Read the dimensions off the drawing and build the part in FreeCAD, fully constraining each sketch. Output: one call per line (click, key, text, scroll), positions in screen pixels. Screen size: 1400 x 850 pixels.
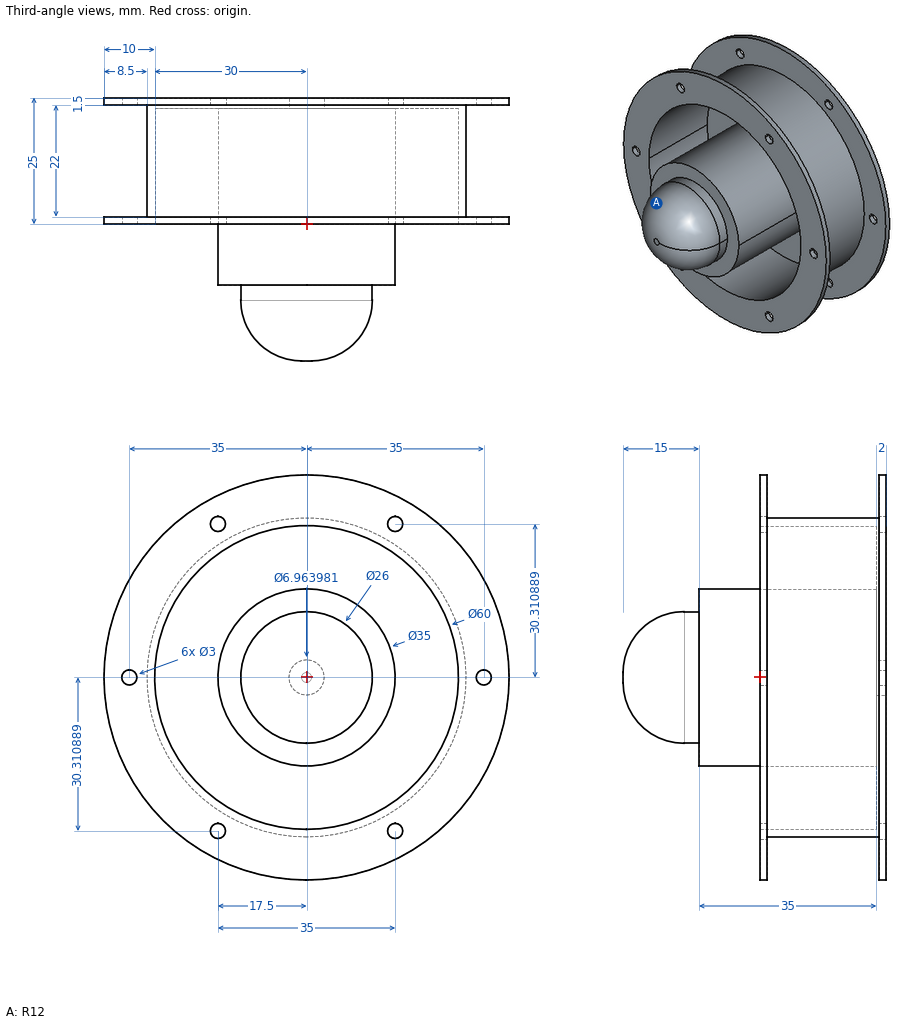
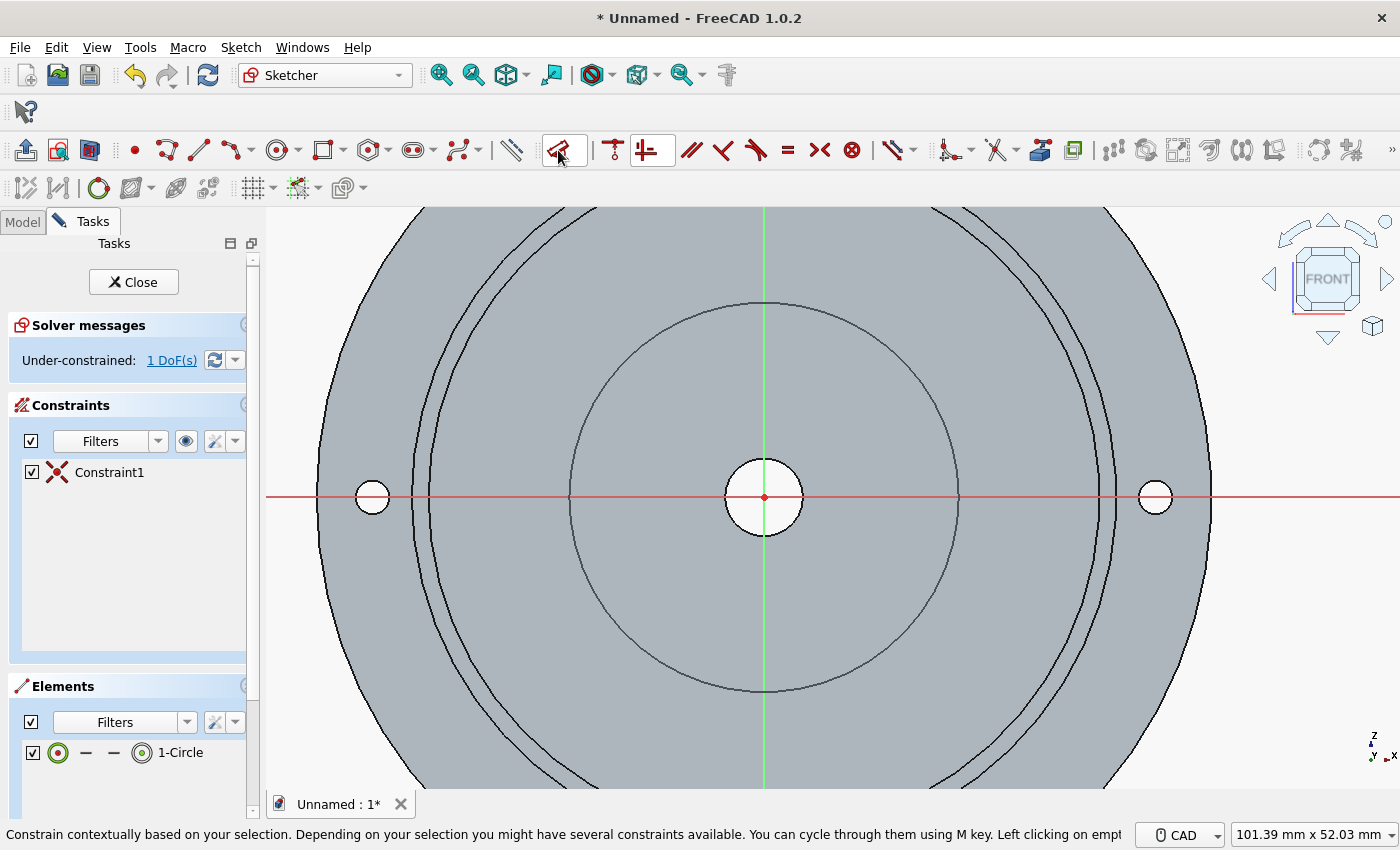
click(901, 359)
click(924, 336)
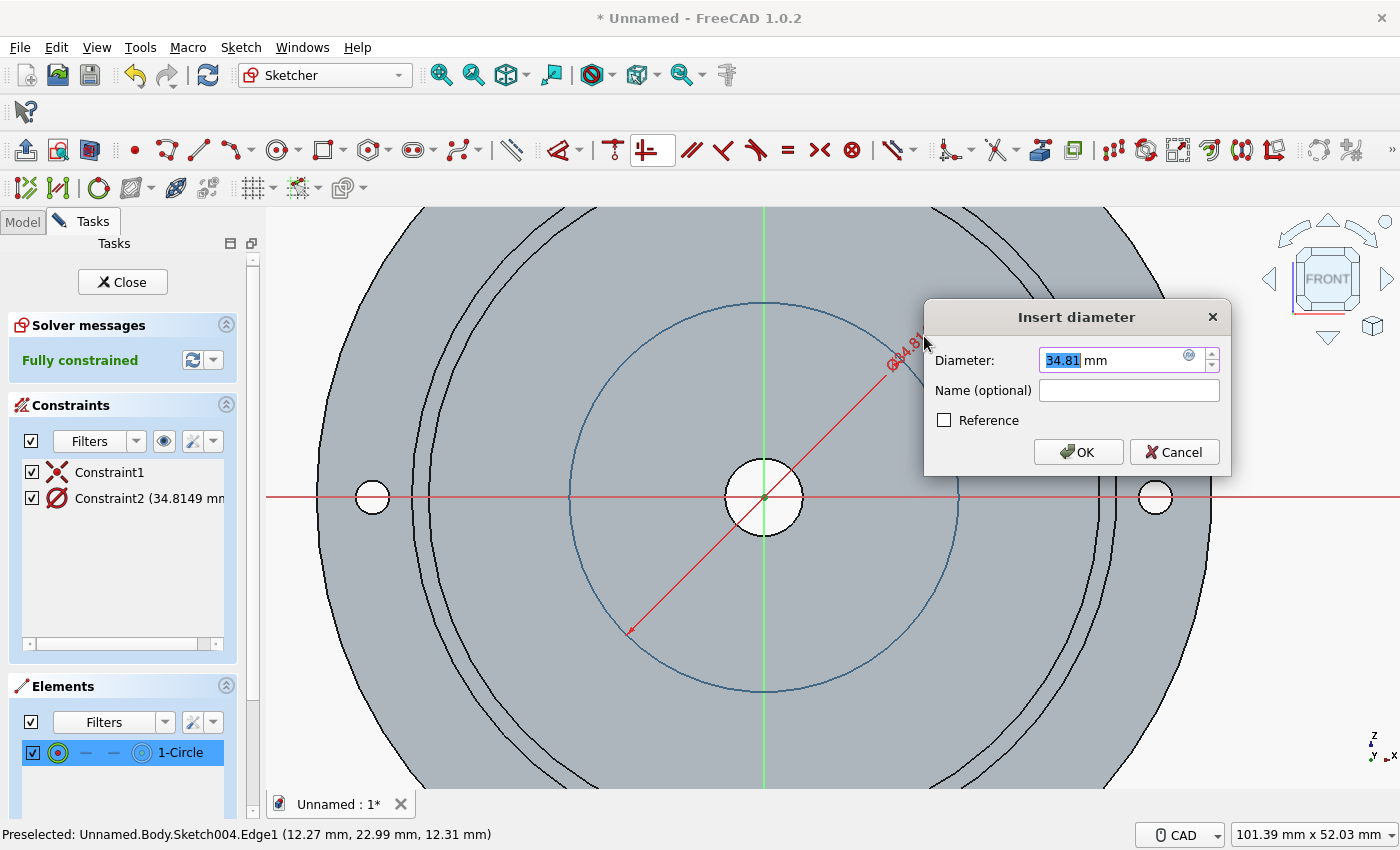
text(35)
key(Return)
key(Escape)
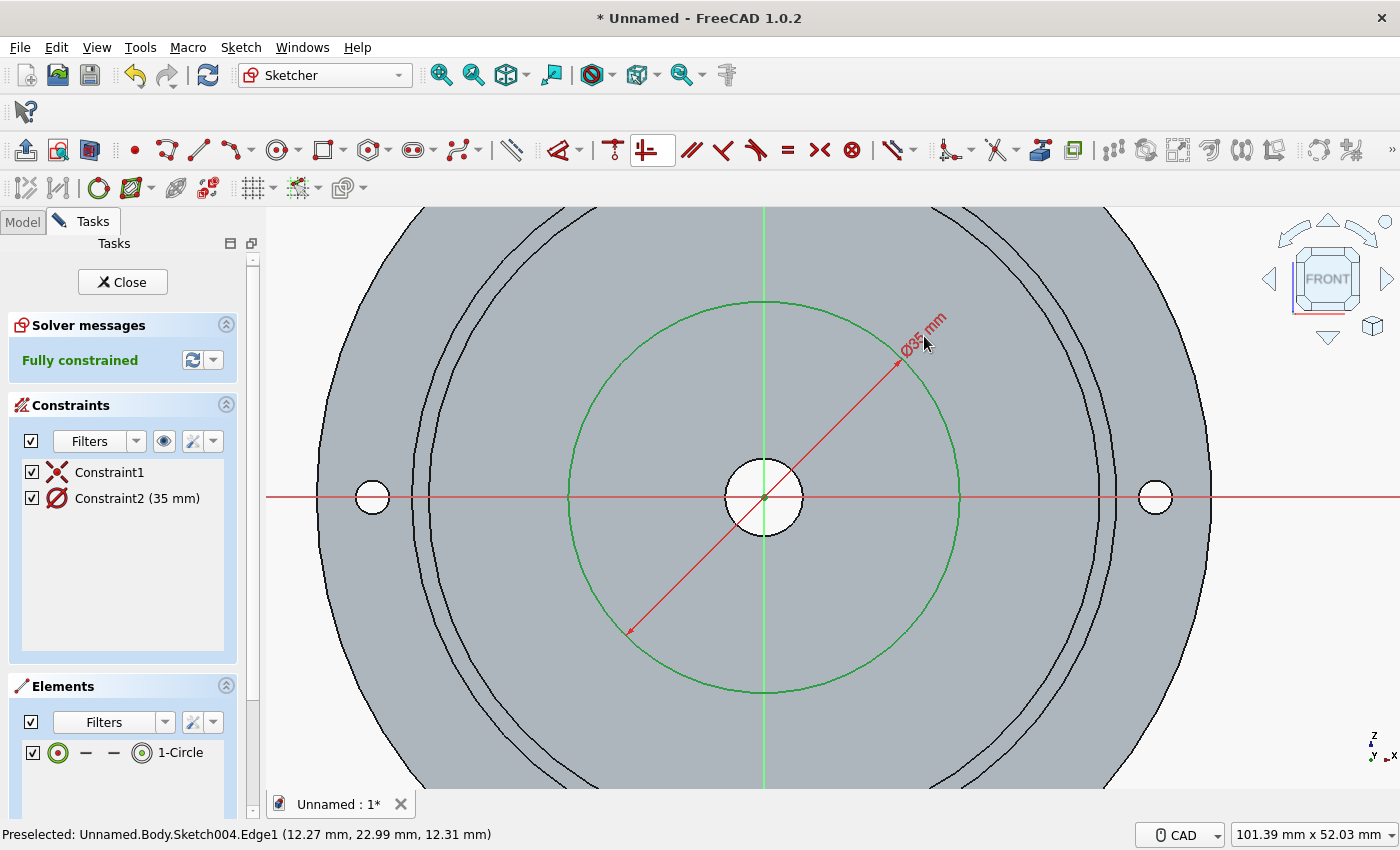
click(123, 282)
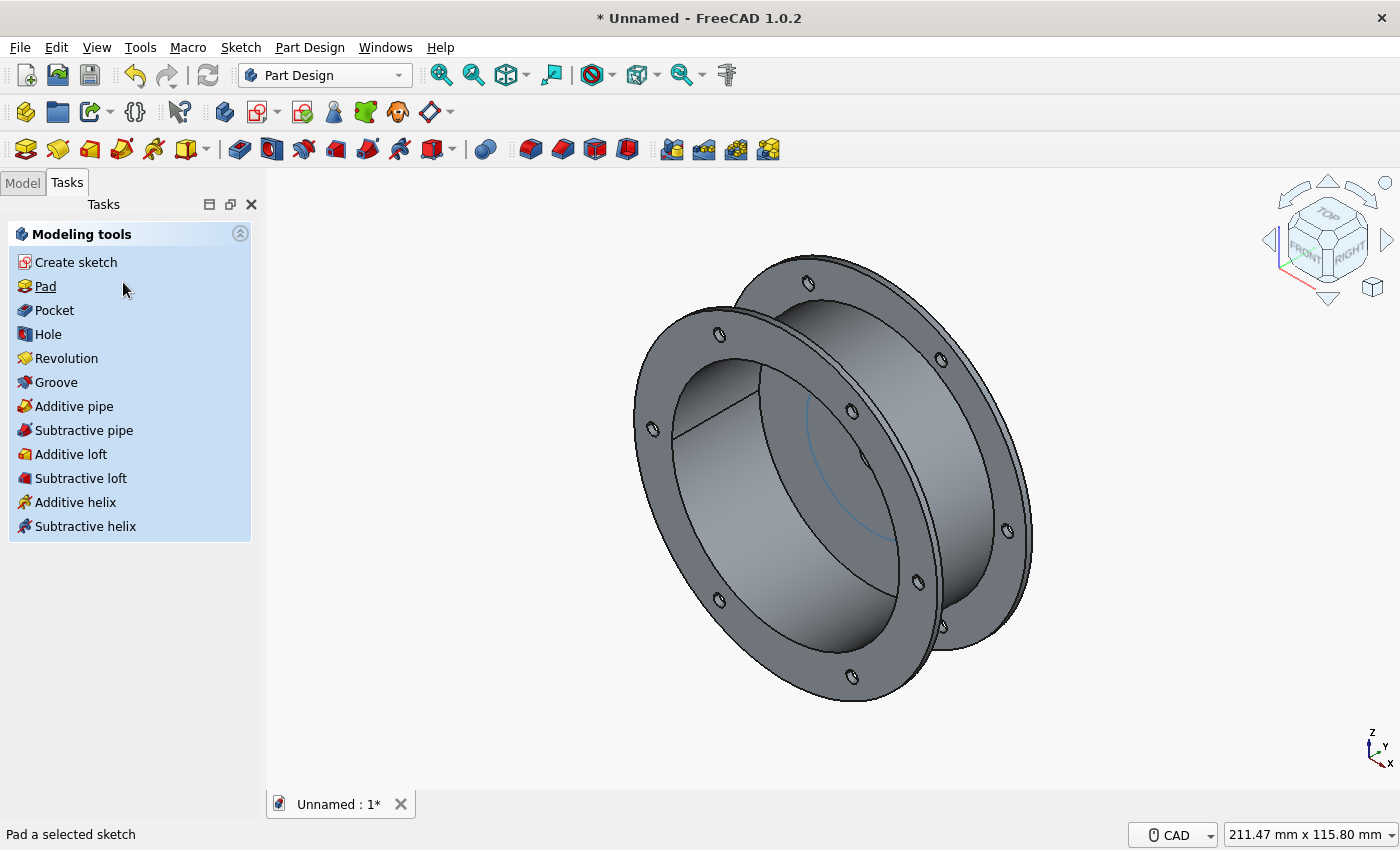
click(26, 150)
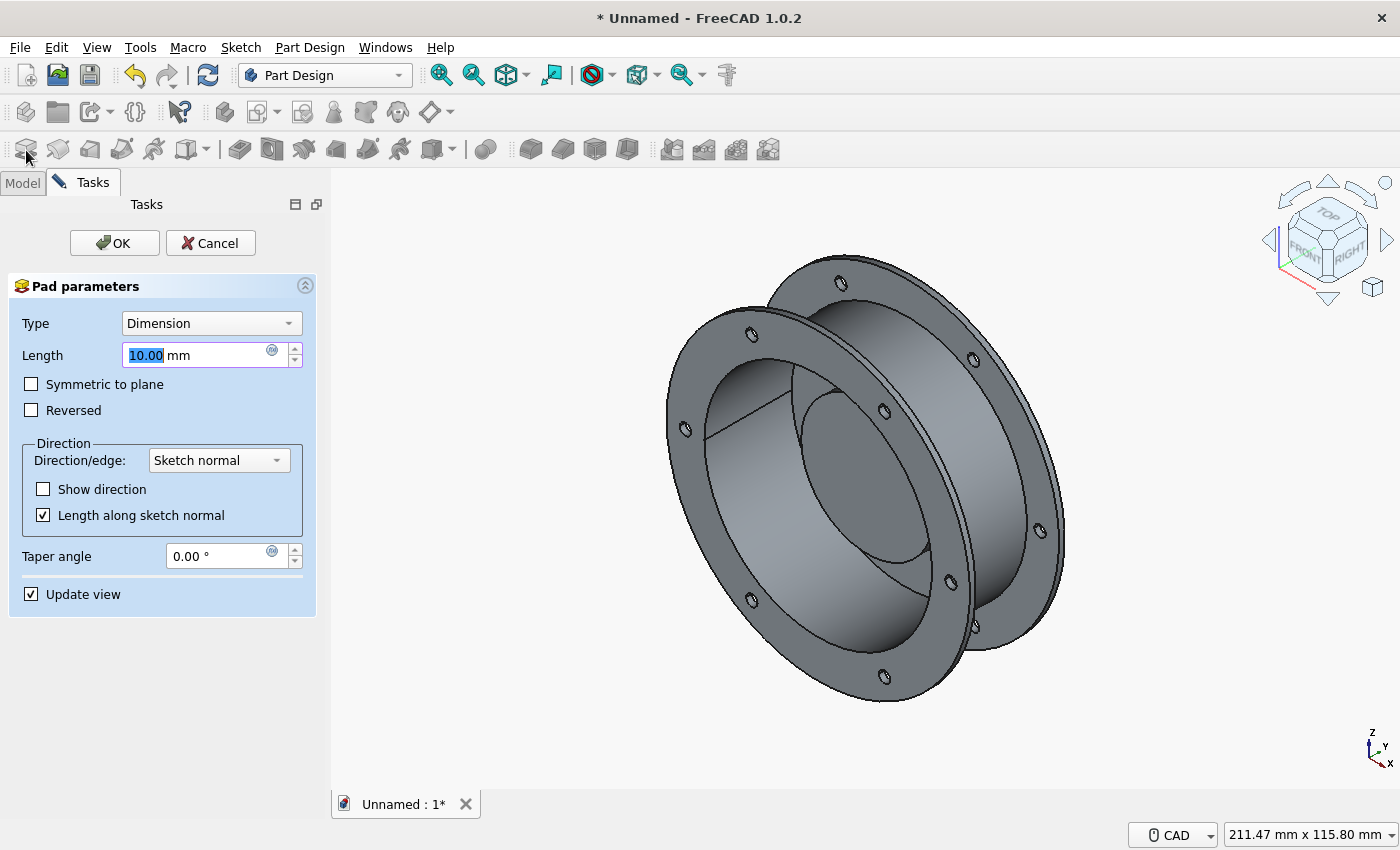
text(35)
key(Tab)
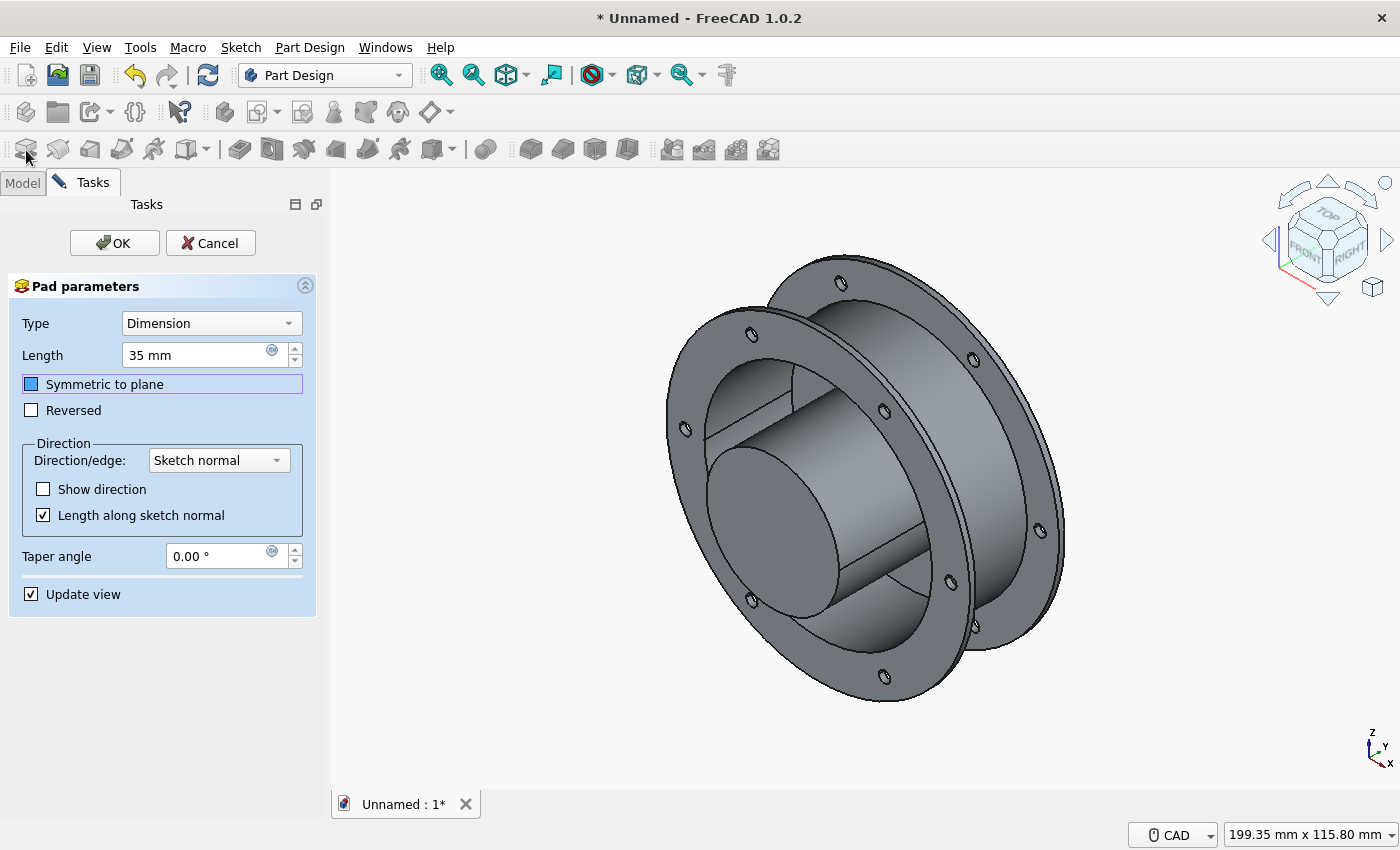
click(115, 243)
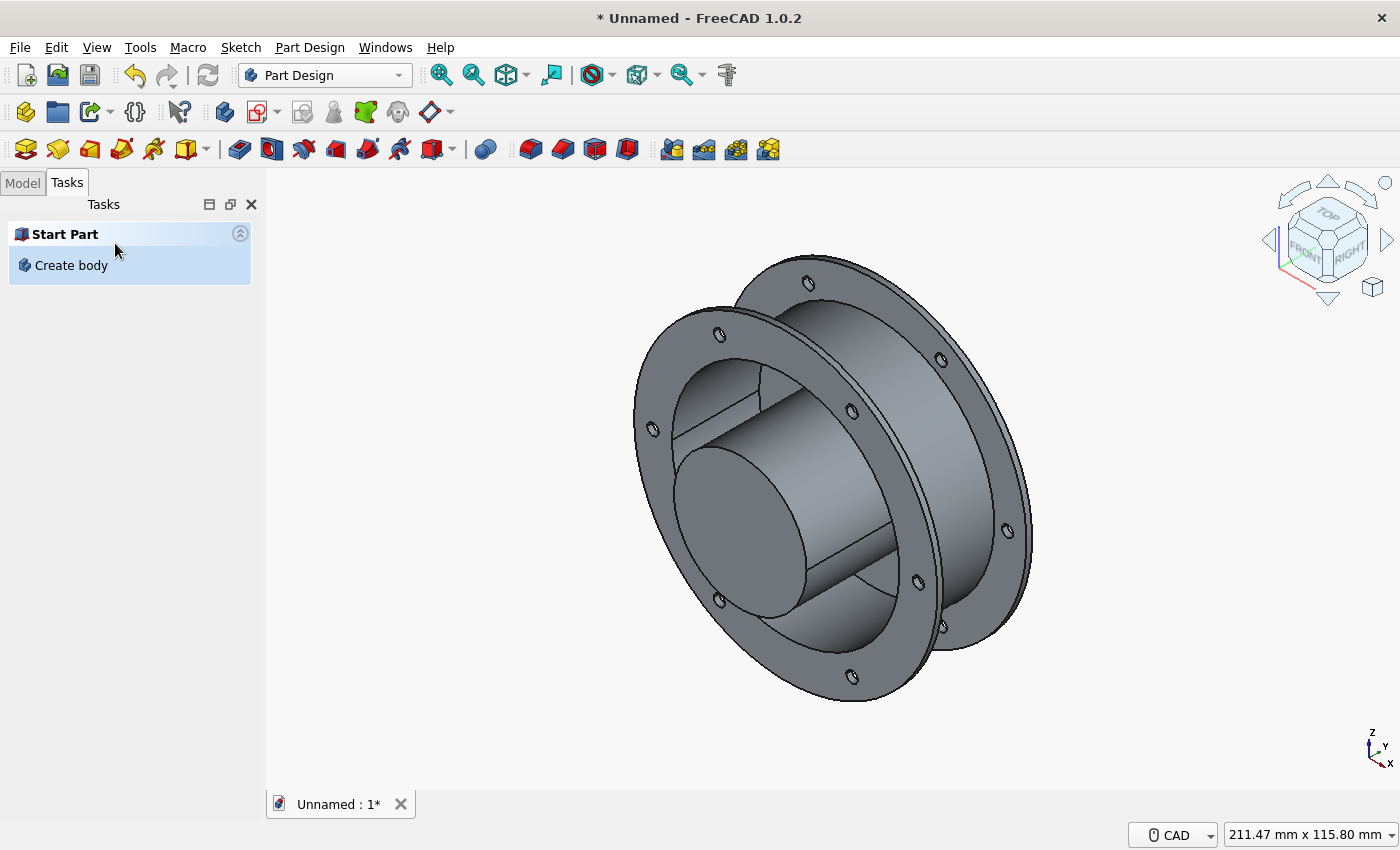
click(442, 76)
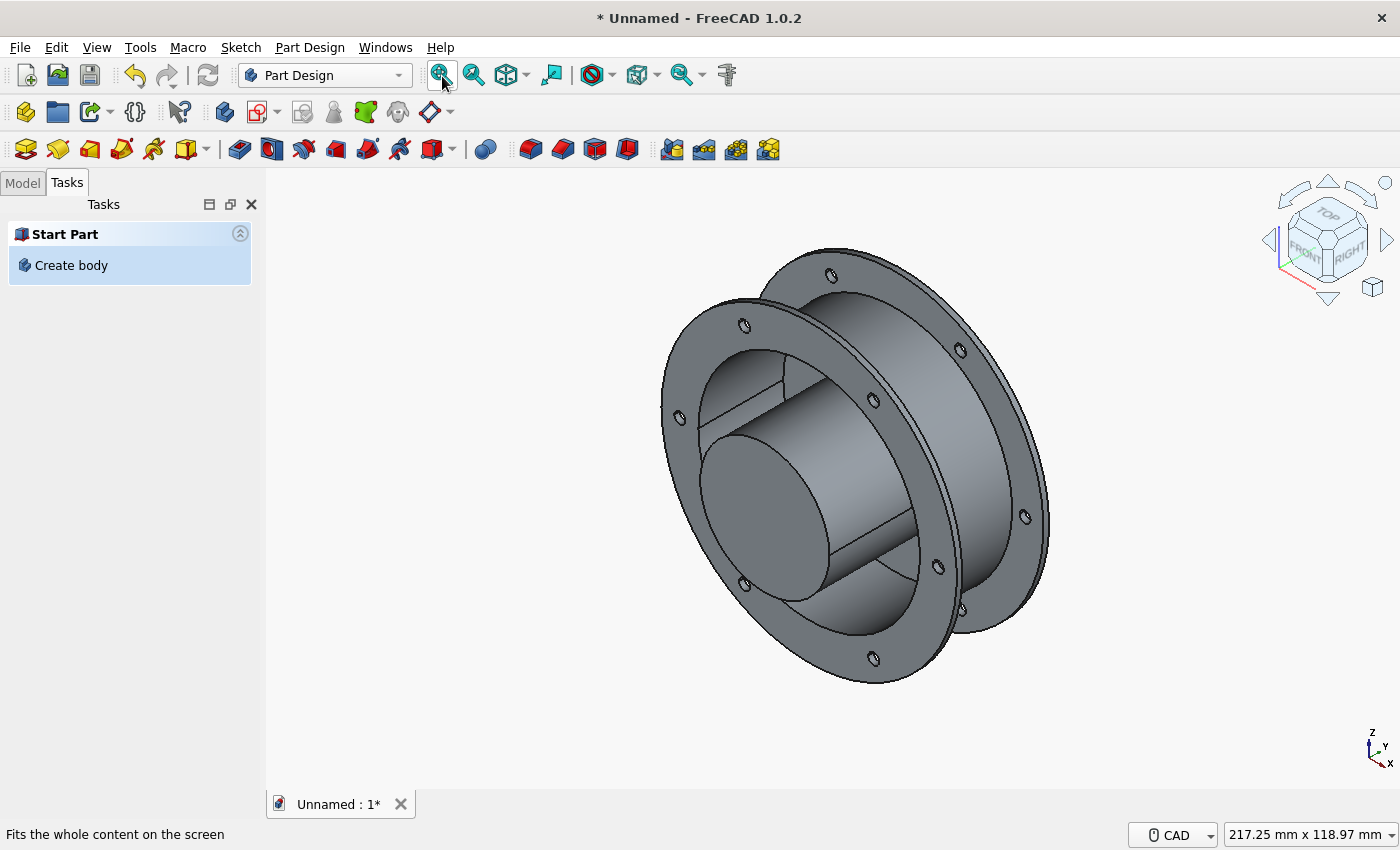
click(765, 517)